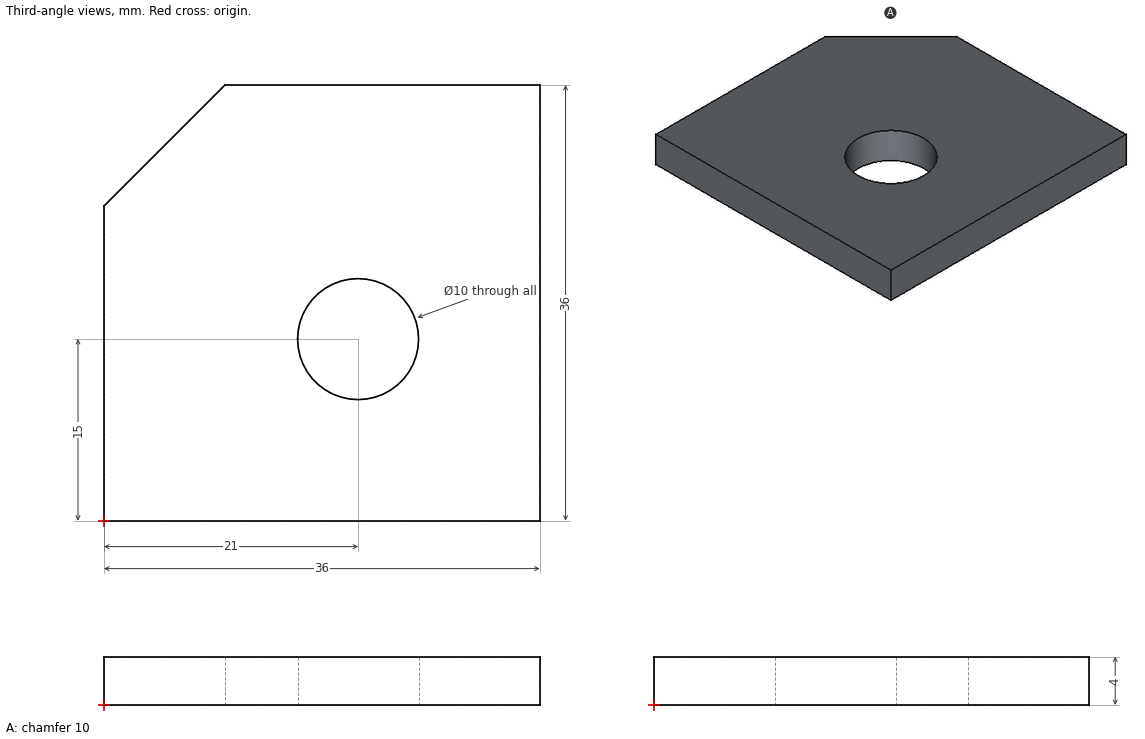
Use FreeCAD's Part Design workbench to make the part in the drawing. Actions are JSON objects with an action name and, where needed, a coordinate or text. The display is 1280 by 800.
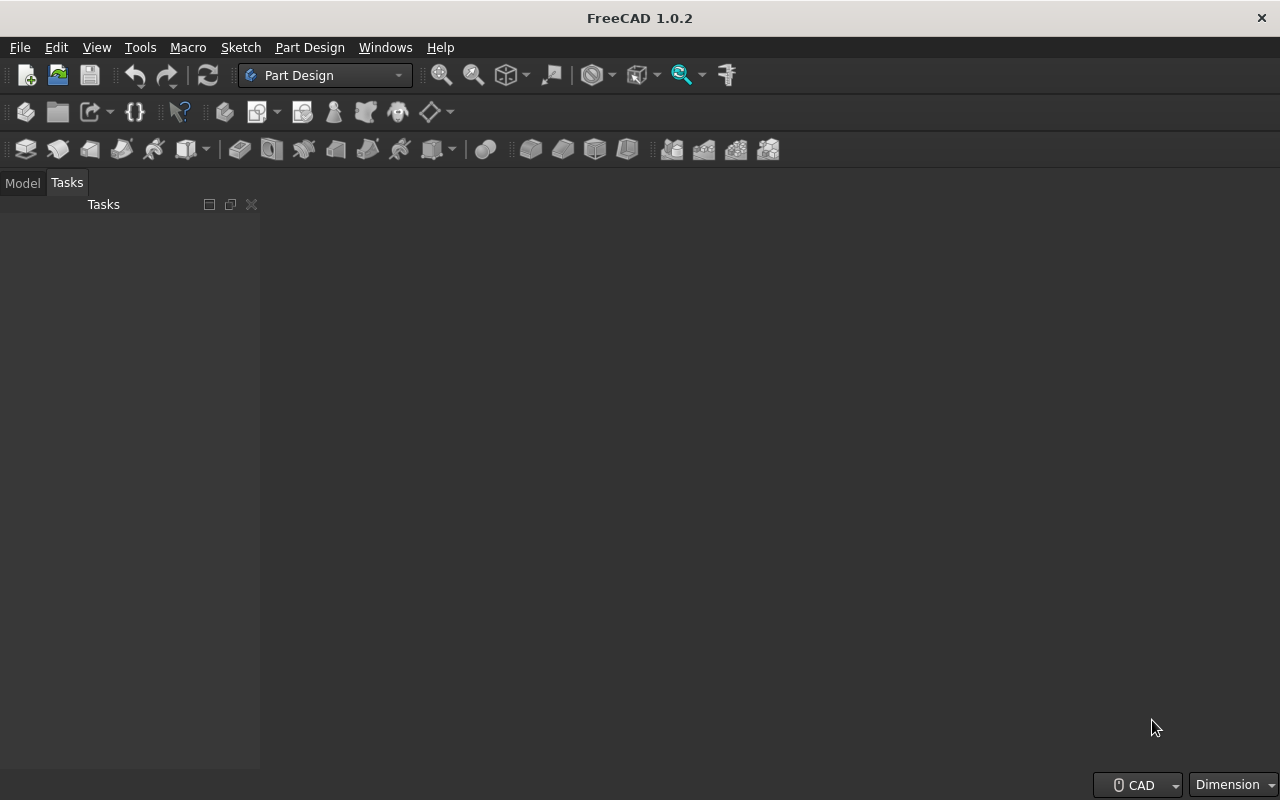
{"action": "key", "text": "ctrl+n"}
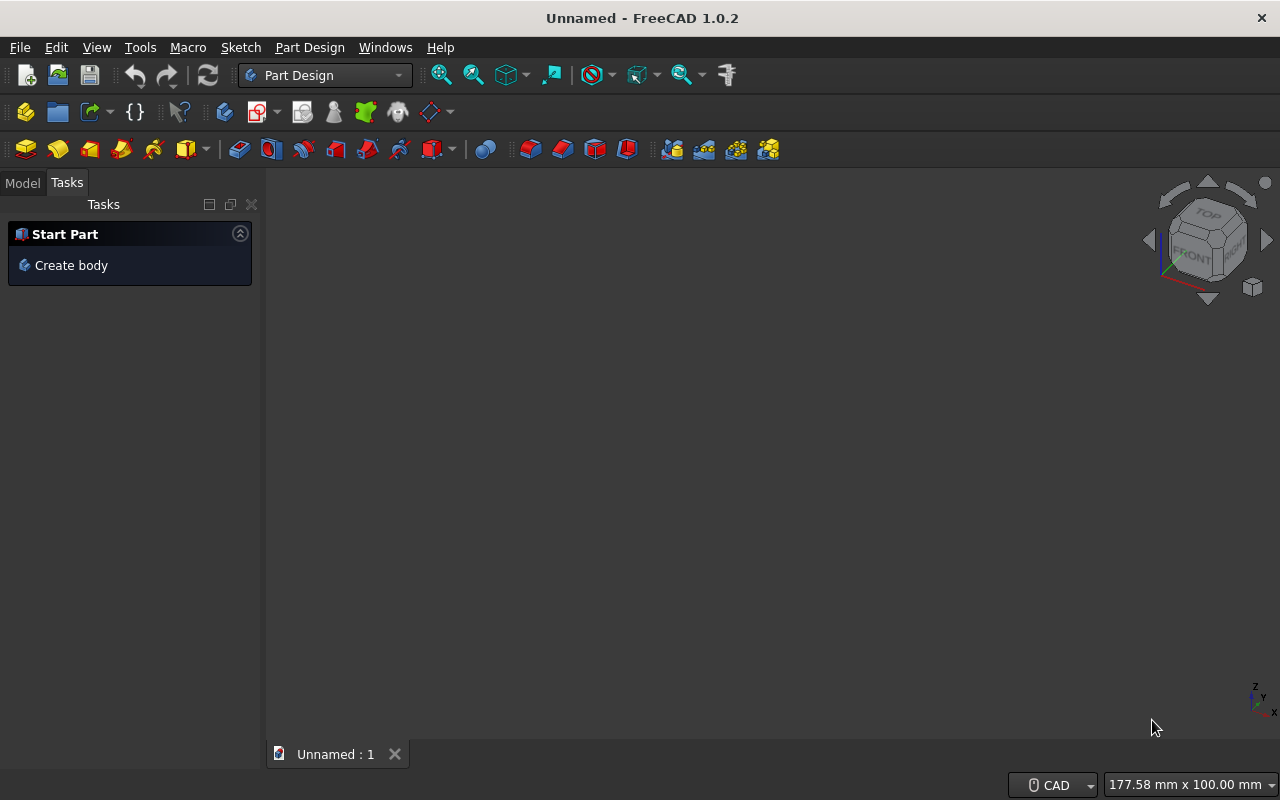
{"action": "left_click", "coordinate": [258, 112]}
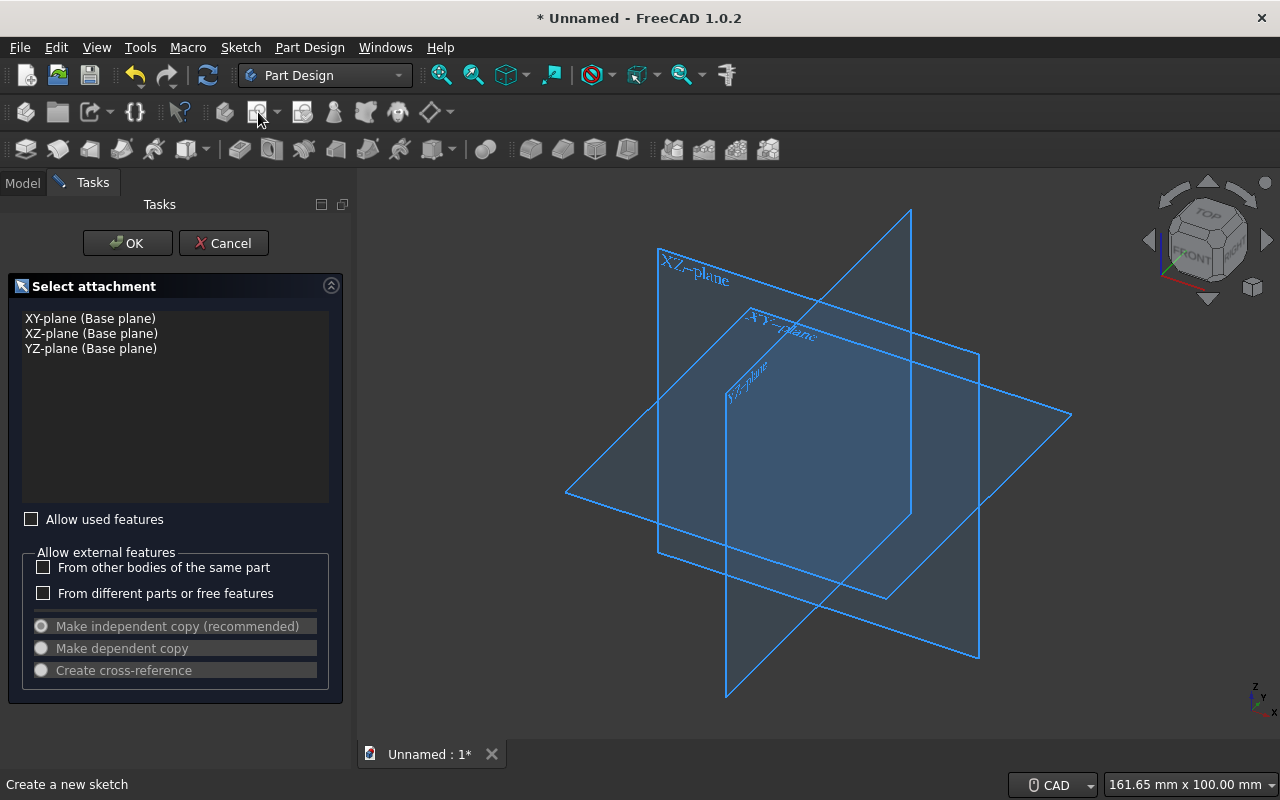
{"action": "left_click", "coordinate": [82, 318]}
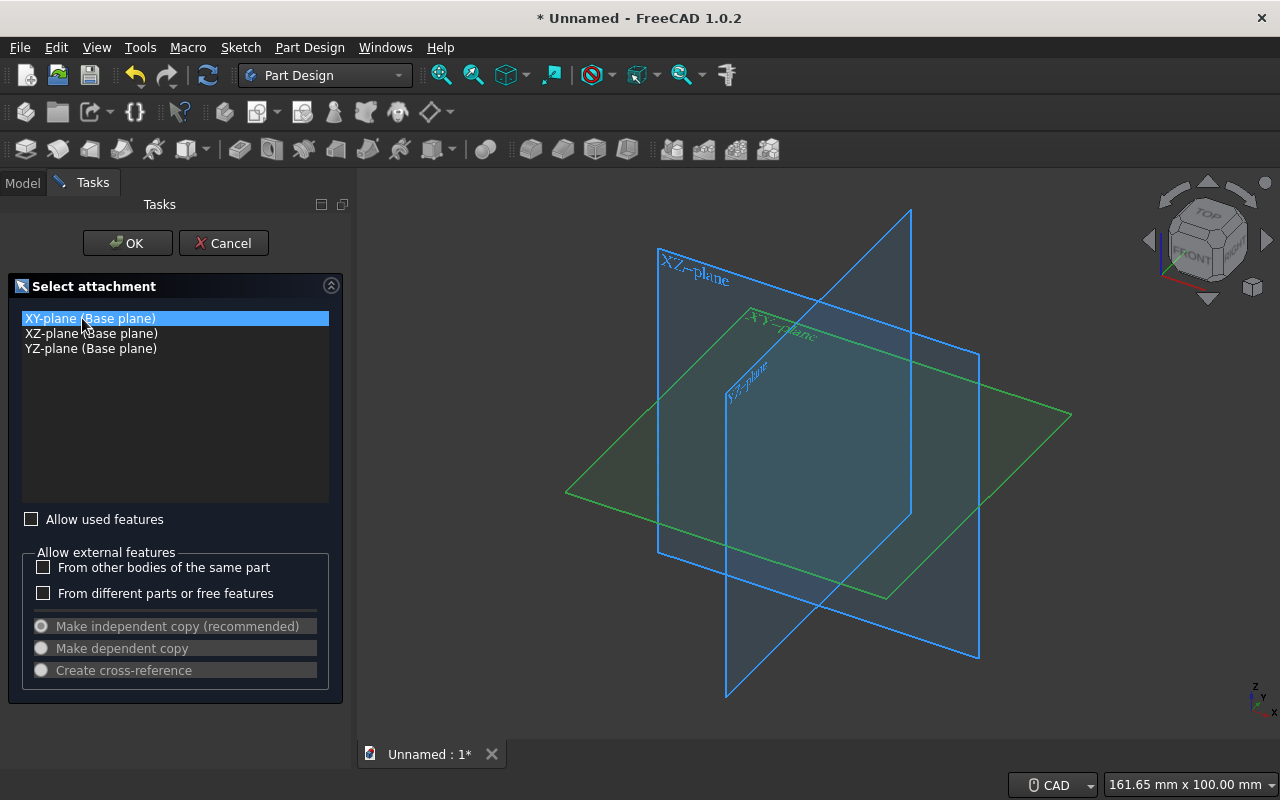
{"action": "left_click", "coordinate": [128, 243]}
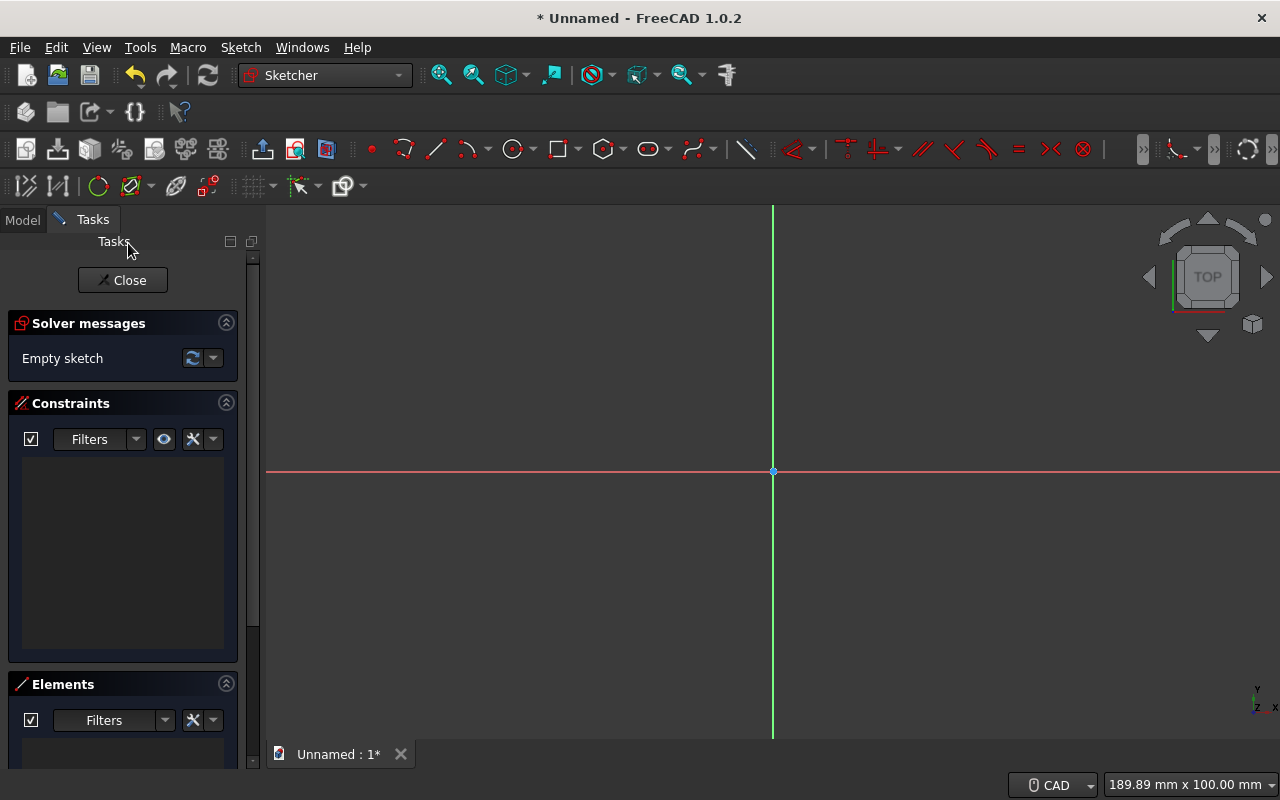
{"action": "scroll", "coordinate": [1069, 259], "scroll_direction": "up", "scroll_amount": 3}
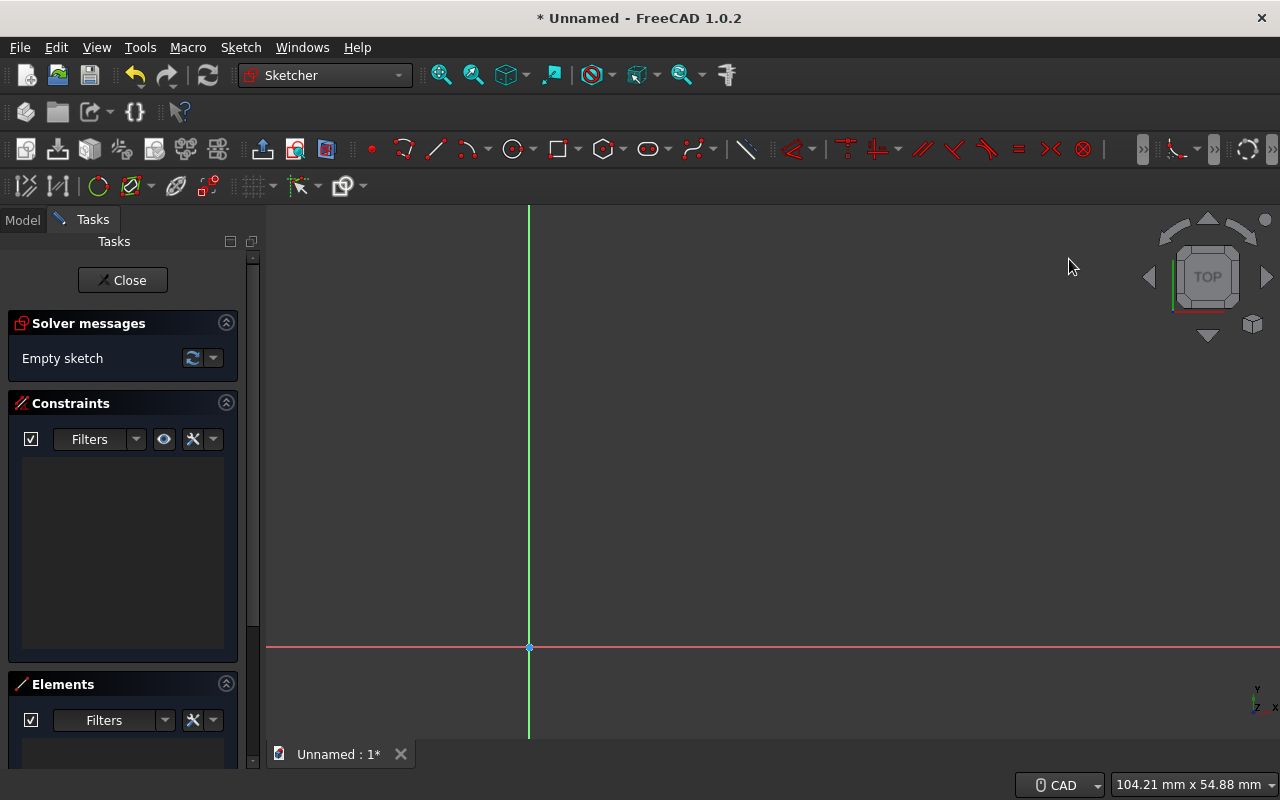
{"action": "key", "text": "g r"}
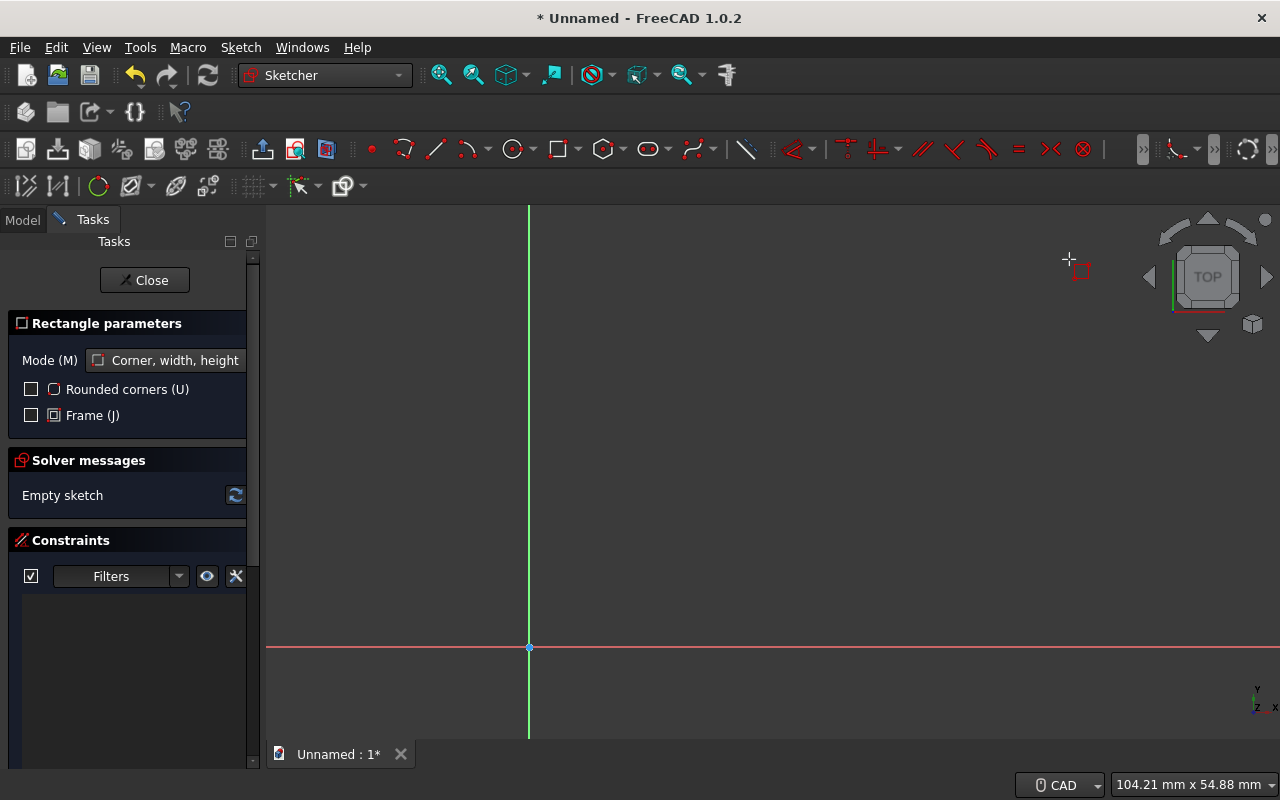
{"action": "left_click", "coordinate": [529, 647]}
{"action": "left_click", "coordinate": [879, 297]}
{"action": "key", "text": "Escape"}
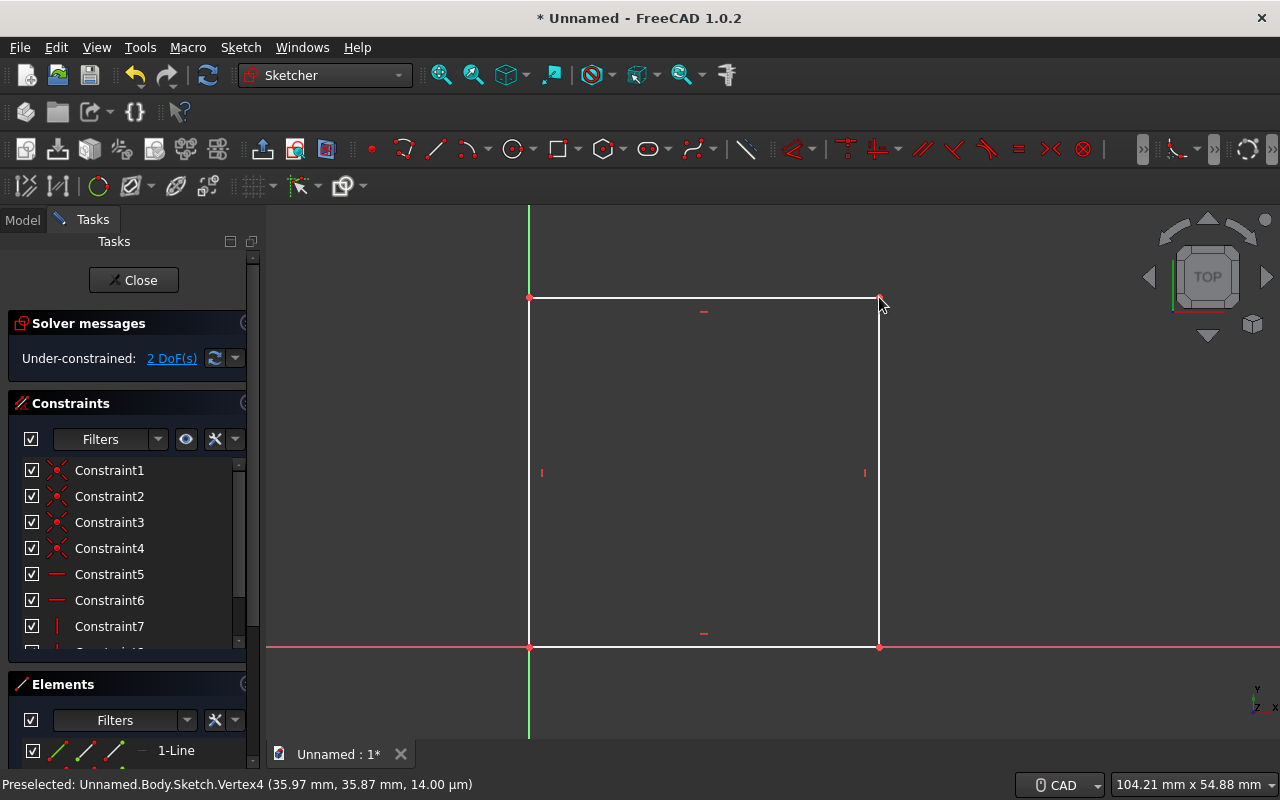
{"action": "key", "text": "d"}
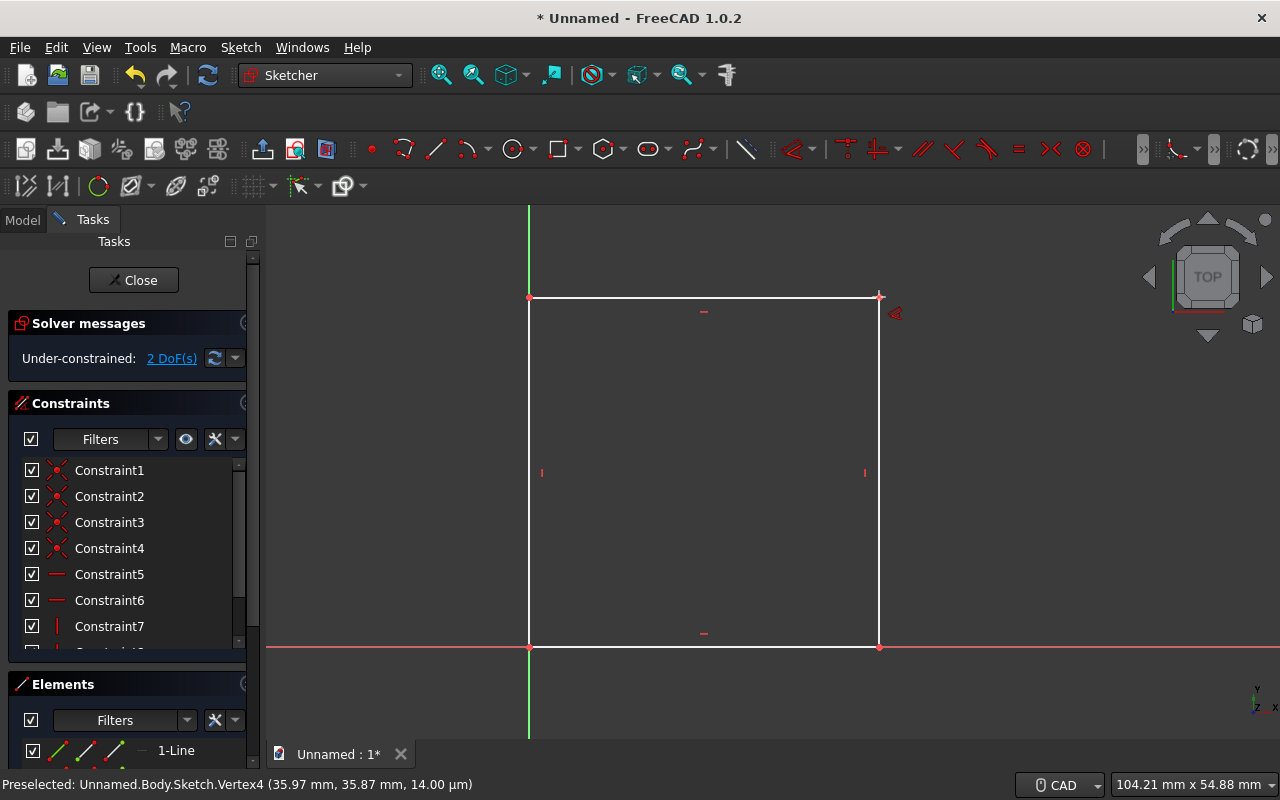
{"action": "left_click", "coordinate": [634, 647]}
{"action": "left_click", "coordinate": [704, 681]}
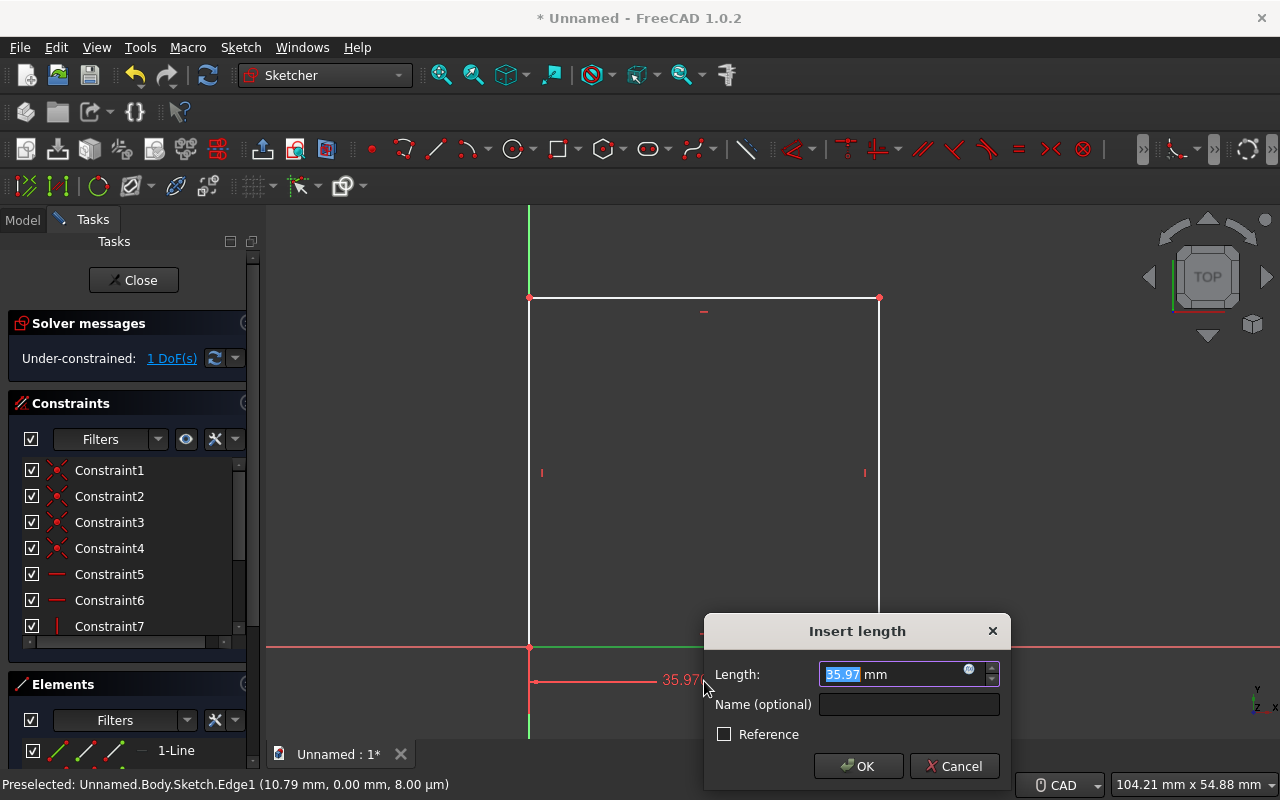
{"action": "type", "text": "36"}
{"action": "key", "text": "Return"}